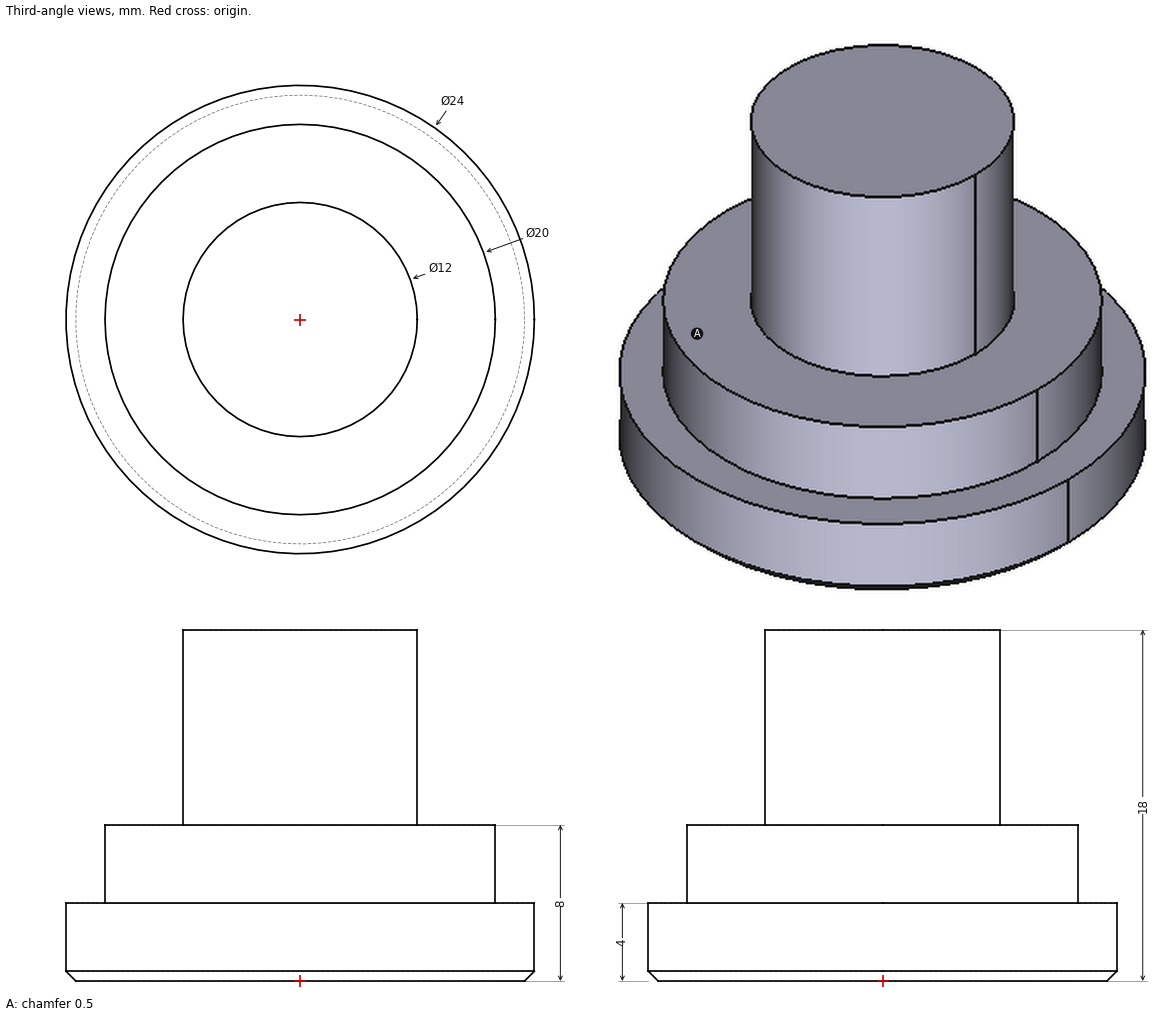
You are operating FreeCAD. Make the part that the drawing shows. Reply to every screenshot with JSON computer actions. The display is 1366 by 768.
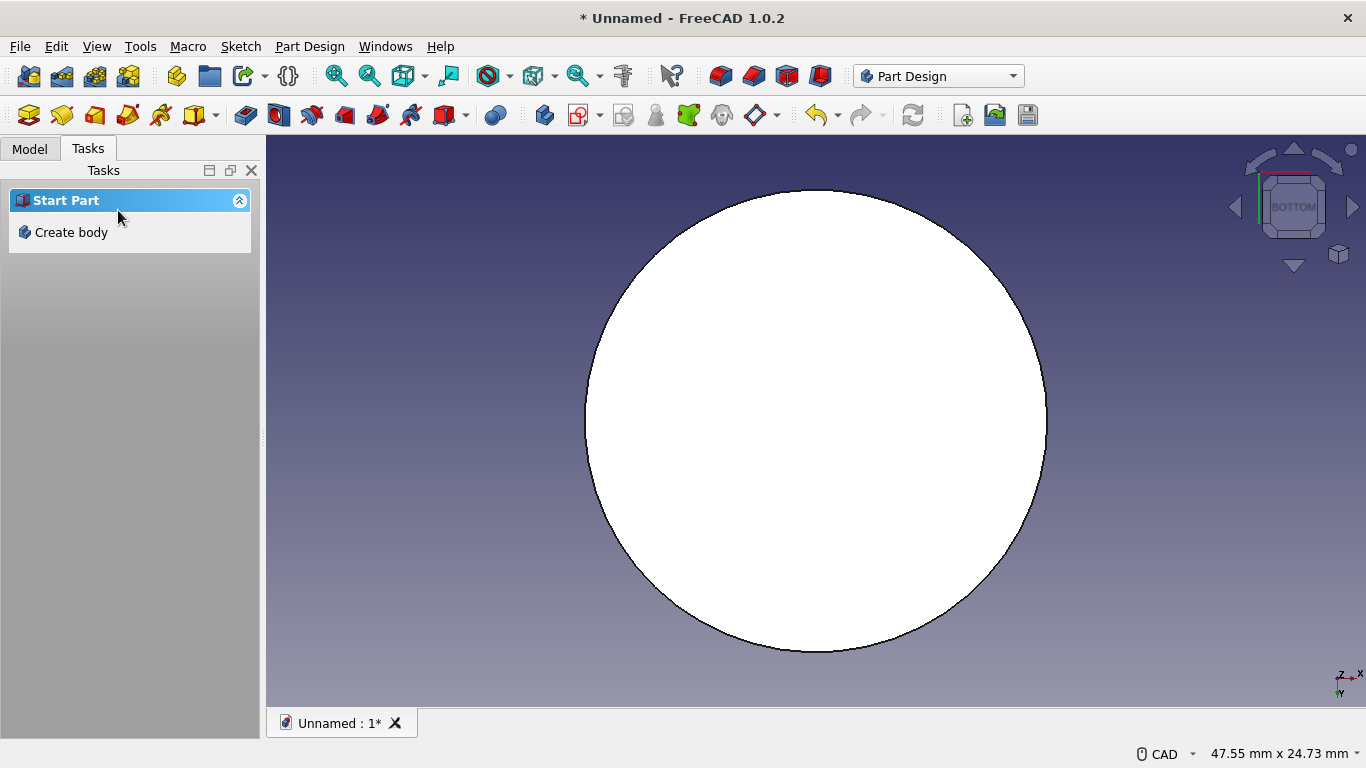
{"action": "left_click", "coordinate": [816, 420]}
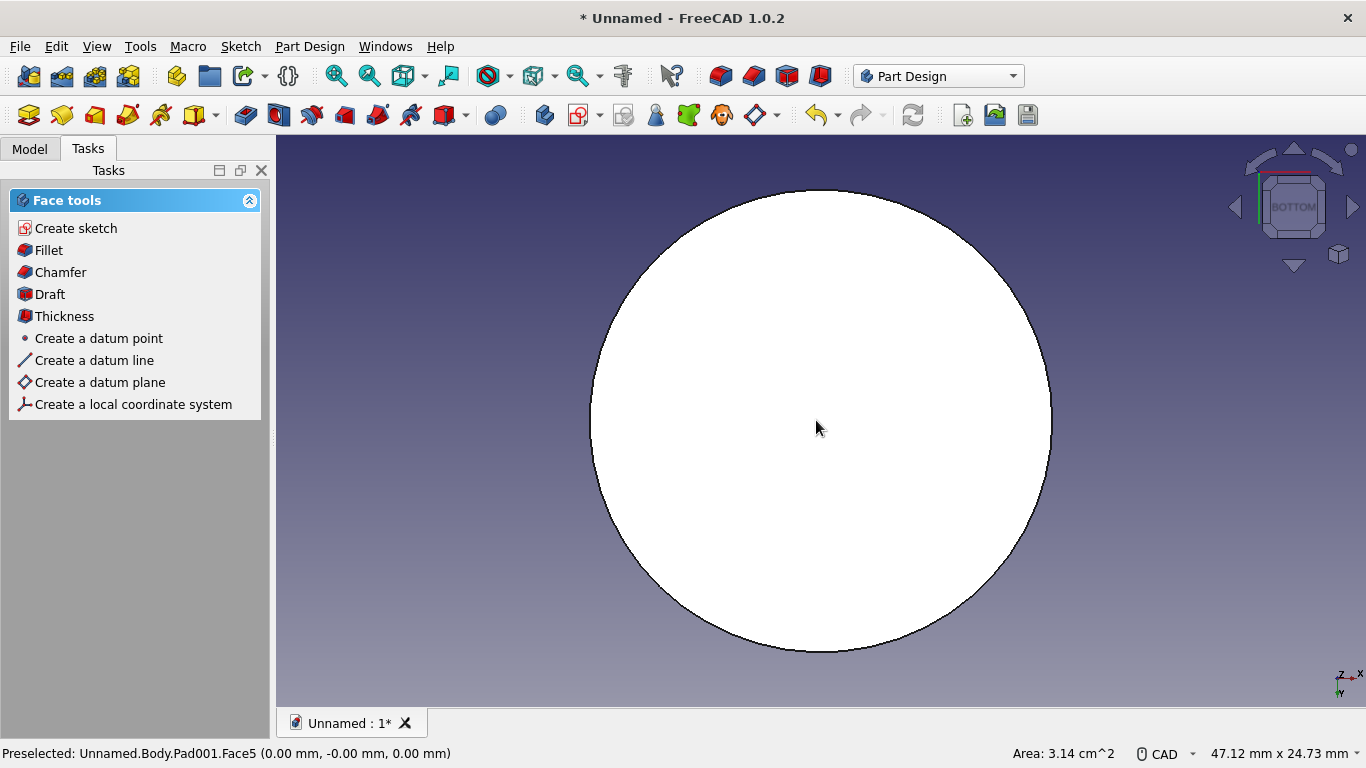
{"action": "left_click", "coordinate": [578, 116]}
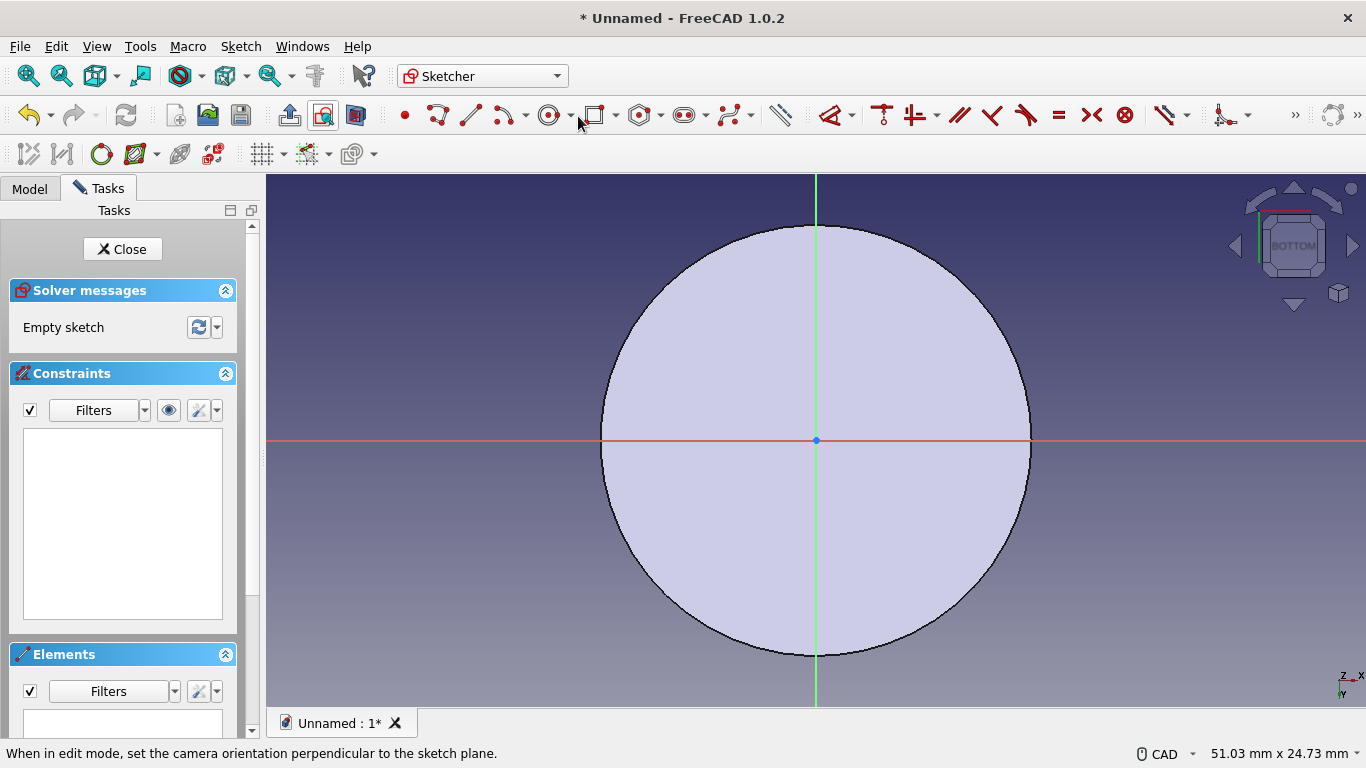
{"action": "scroll", "coordinate": [608, 440], "scroll_direction": "down", "scroll_amount": 2}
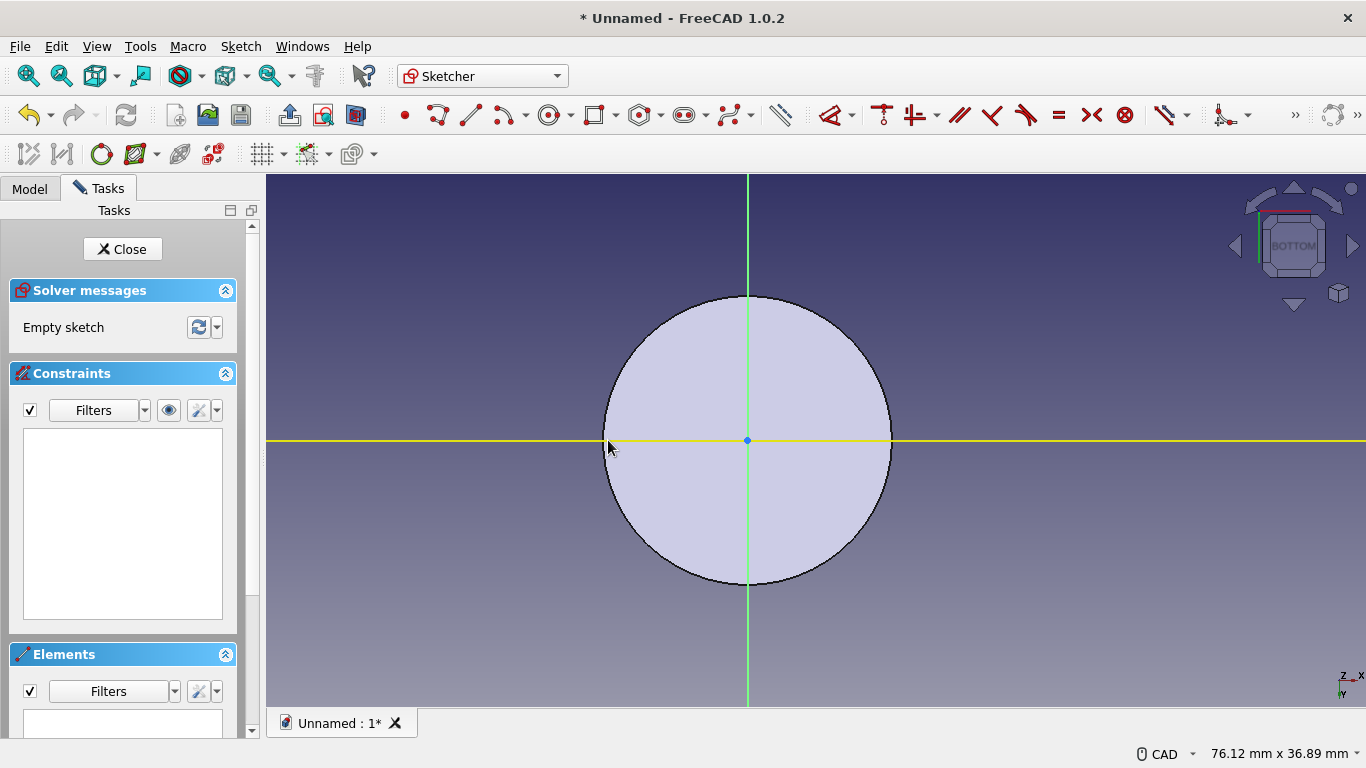
{"action": "left_click", "coordinate": [548, 116]}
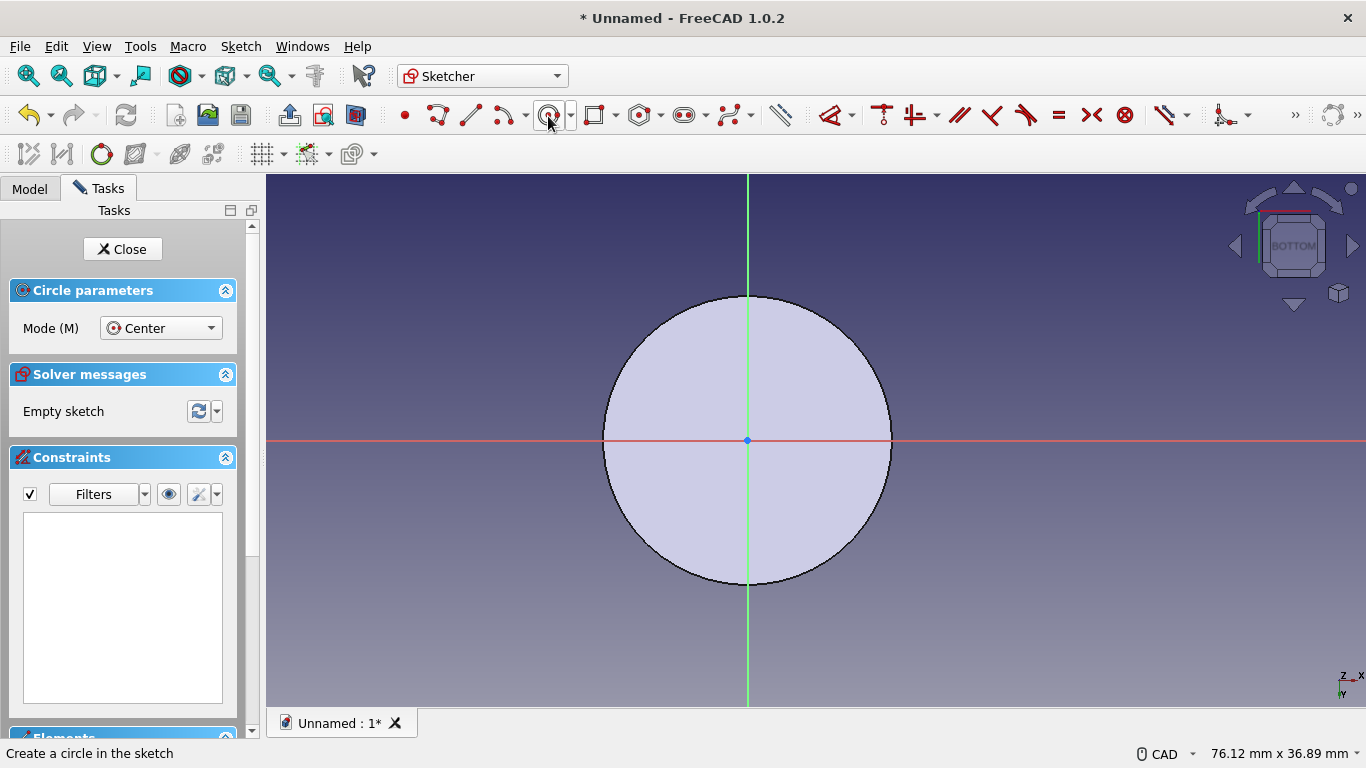
{"action": "left_click", "coordinate": [748, 441]}
{"action": "mouse_move", "coordinate": [870, 318]}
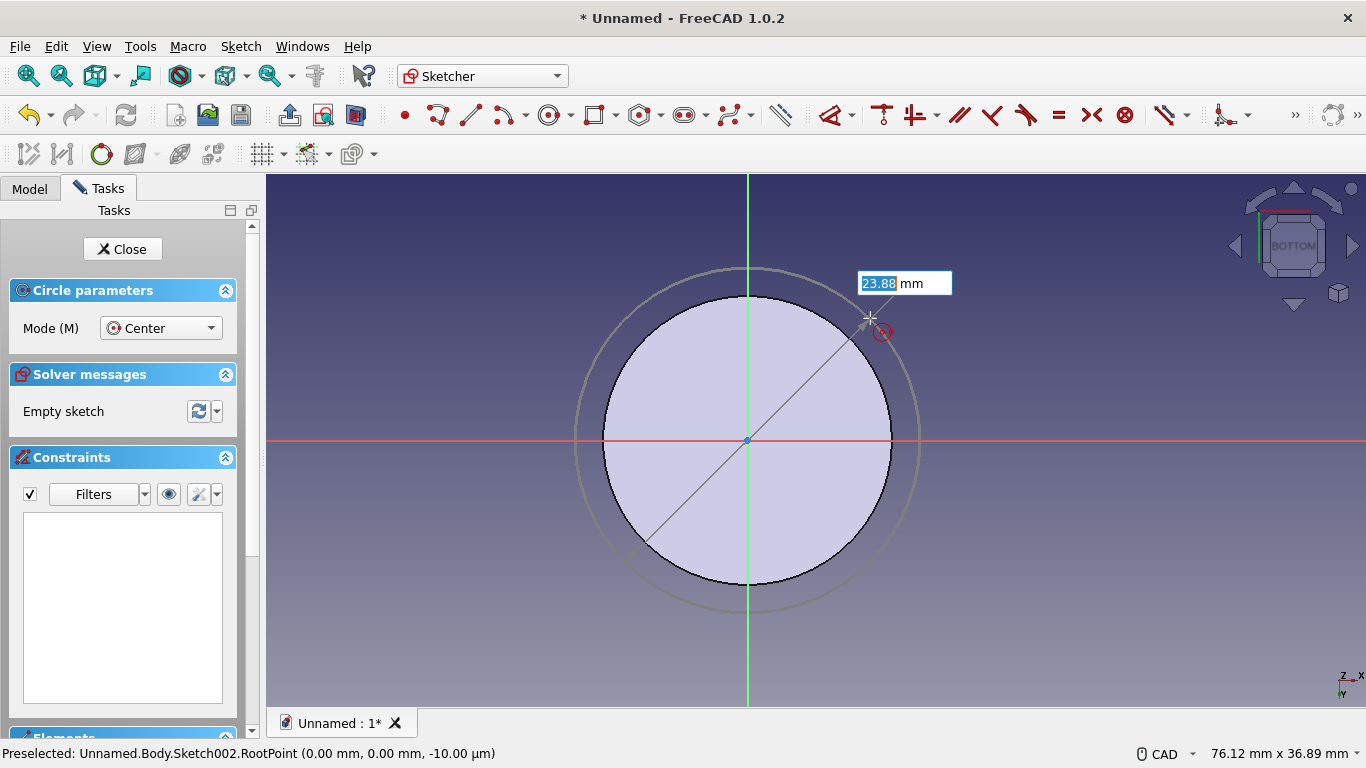
{"action": "type", "text": "24"}
{"action": "key", "text": "Return"}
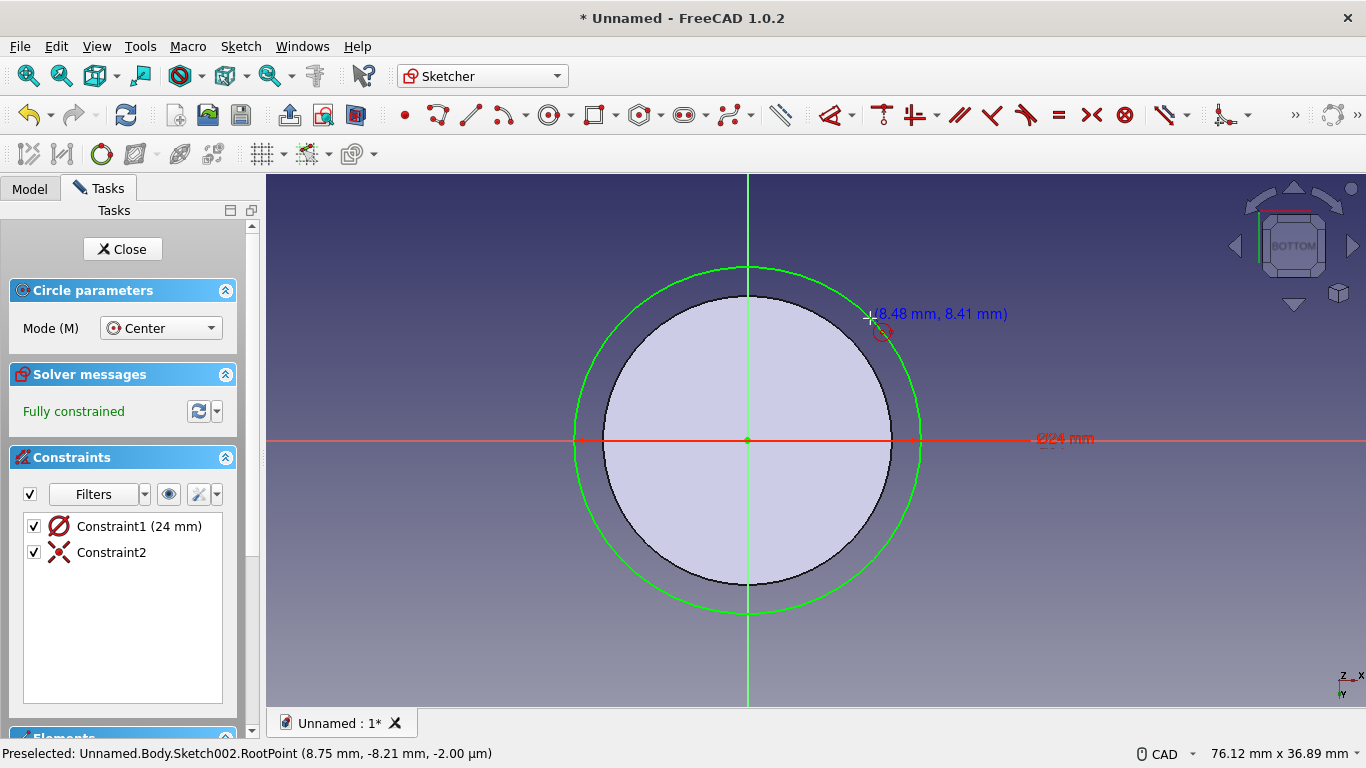
{"action": "left_click", "coordinate": [748, 441]}
{"action": "mouse_move", "coordinate": [850, 338]}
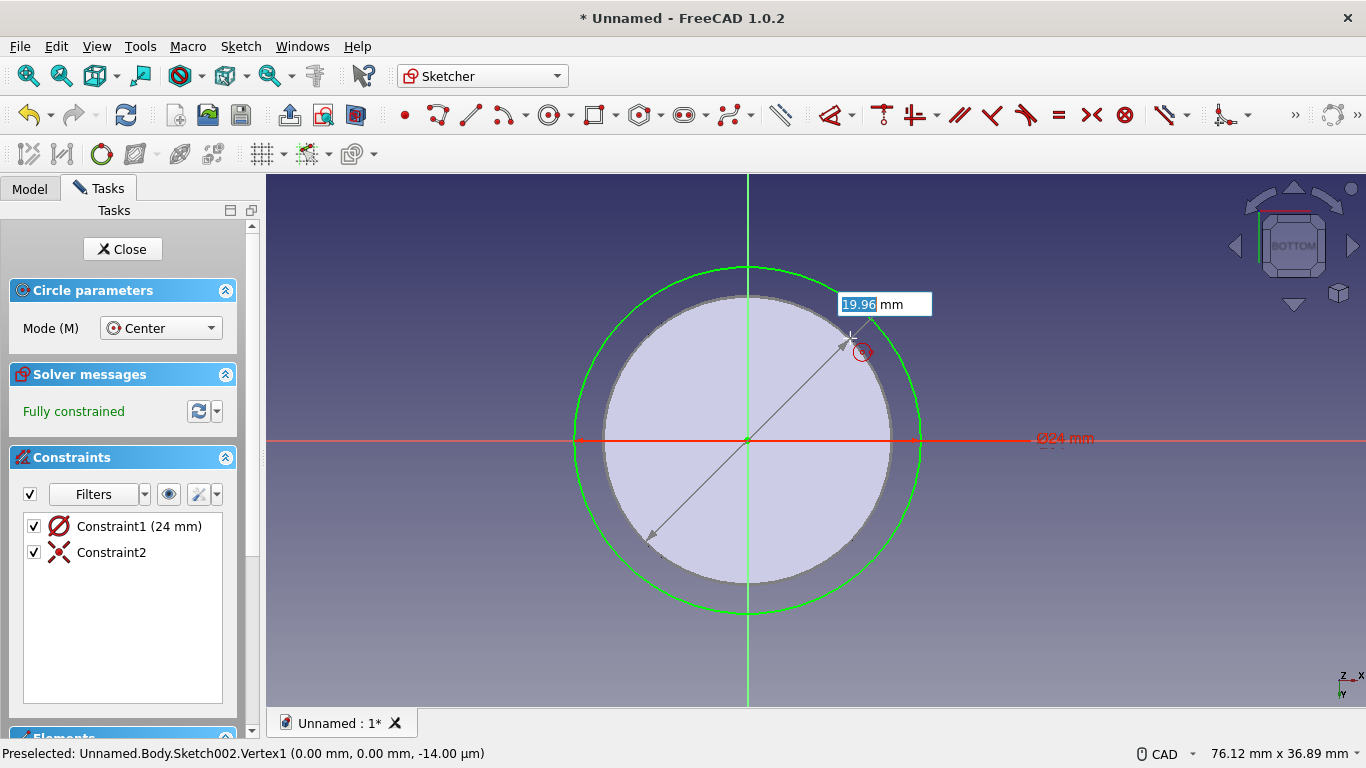
{"action": "type", "text": "20"}
{"action": "key", "text": "Return"}
{"action": "key", "text": "Escape"}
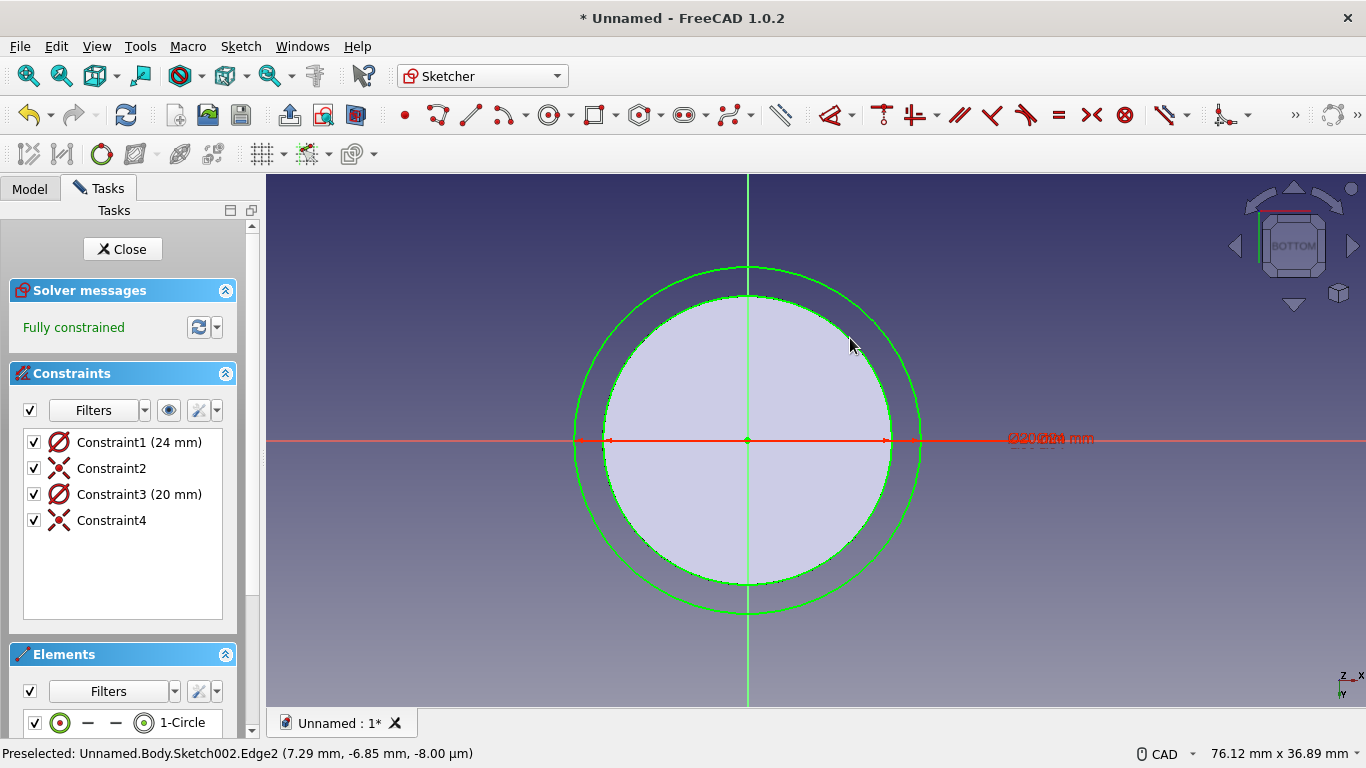
{"action": "left_click", "coordinate": [123, 249]}